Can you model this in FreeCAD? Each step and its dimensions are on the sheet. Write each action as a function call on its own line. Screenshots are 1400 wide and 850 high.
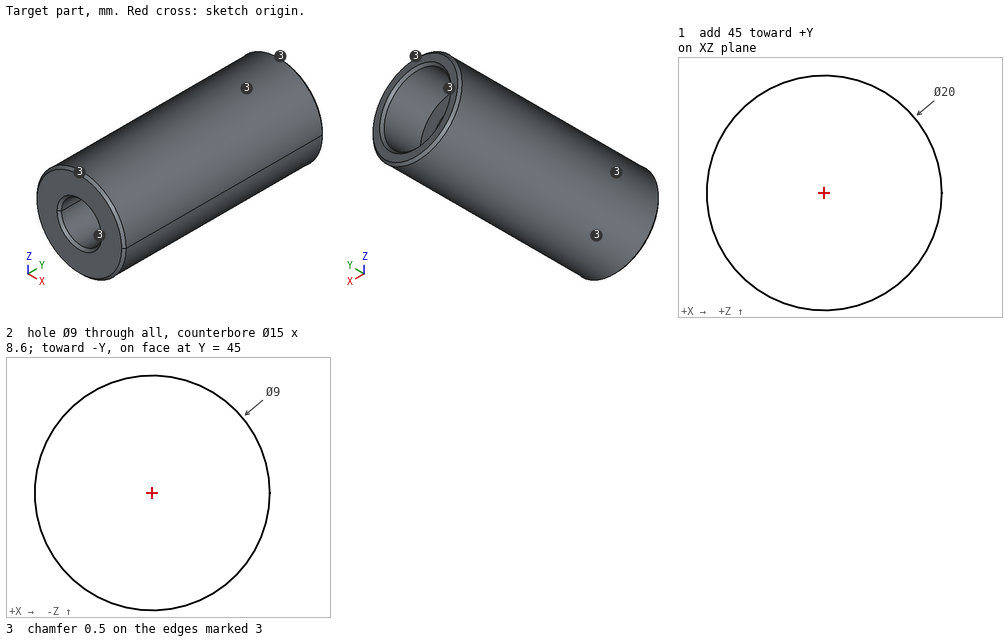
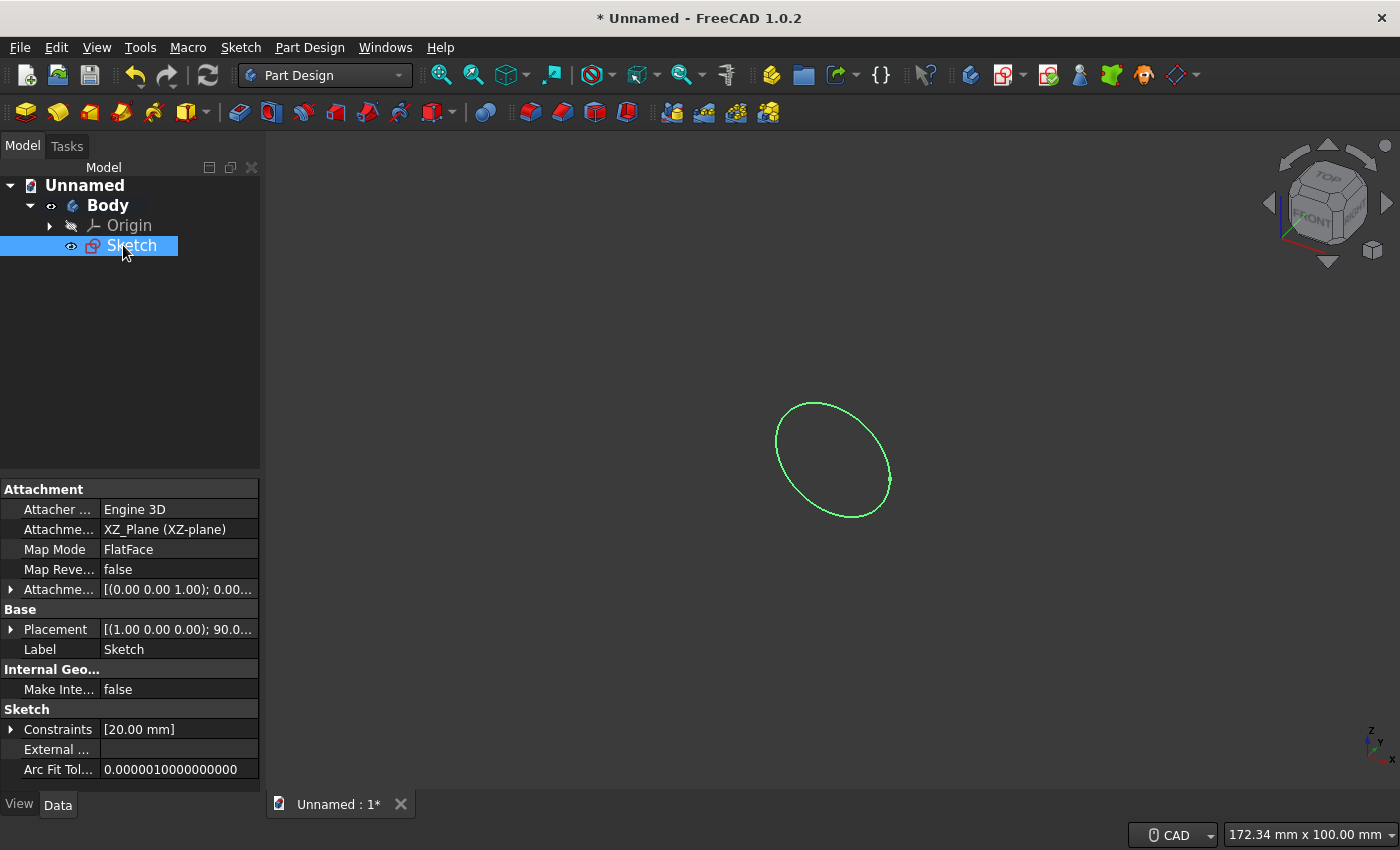
click(26, 112)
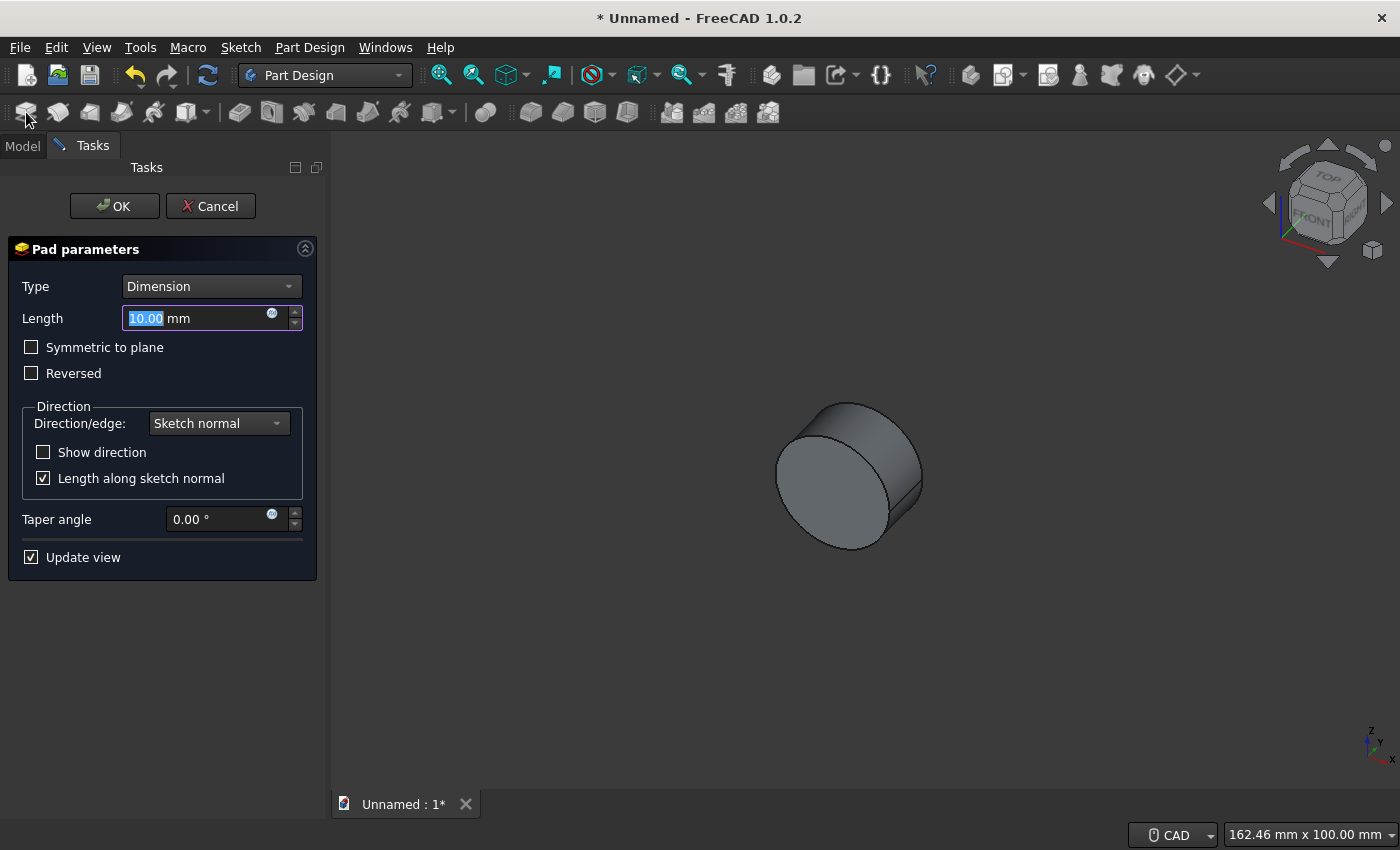
text(45)
key(Tab)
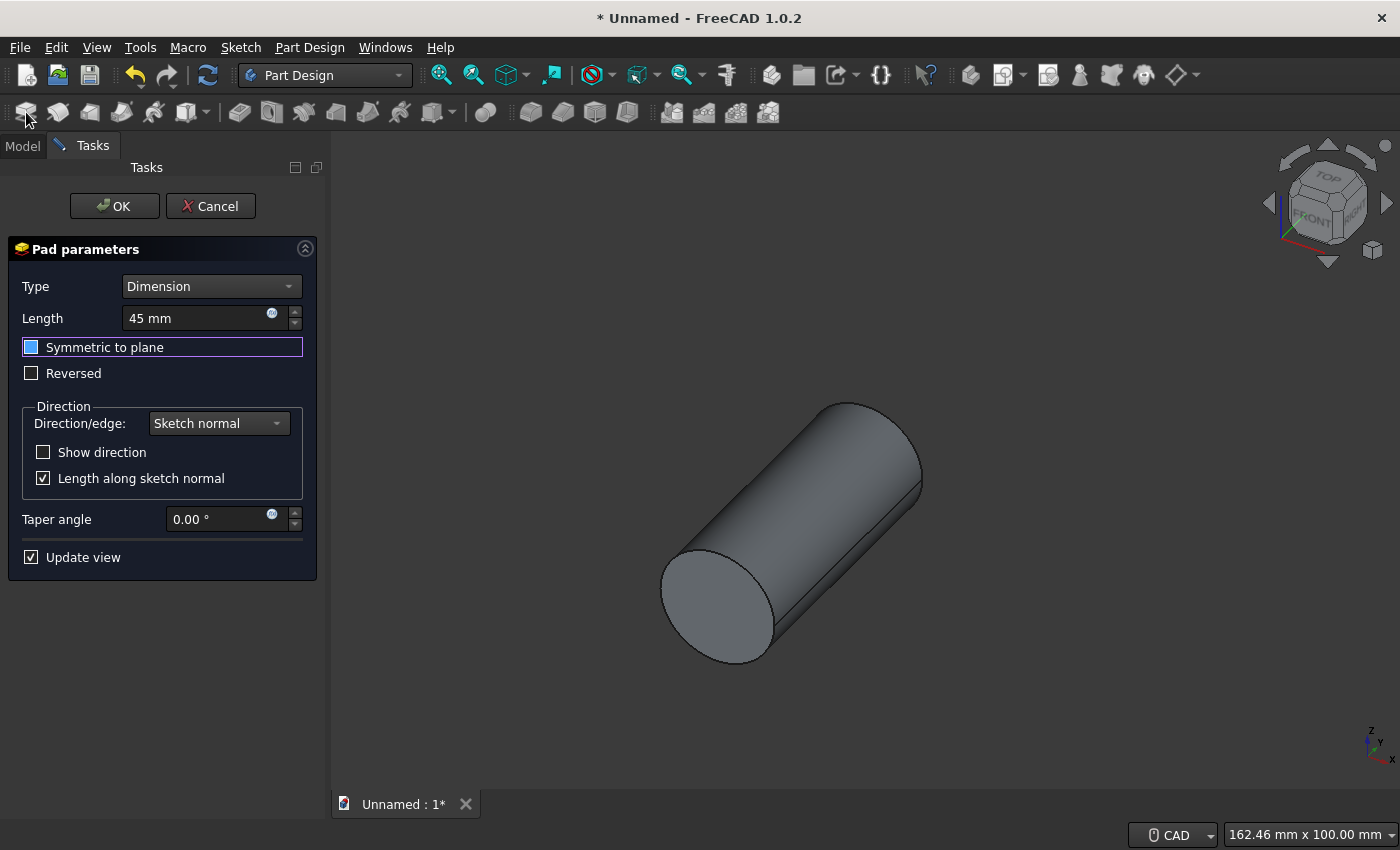
click(30, 373)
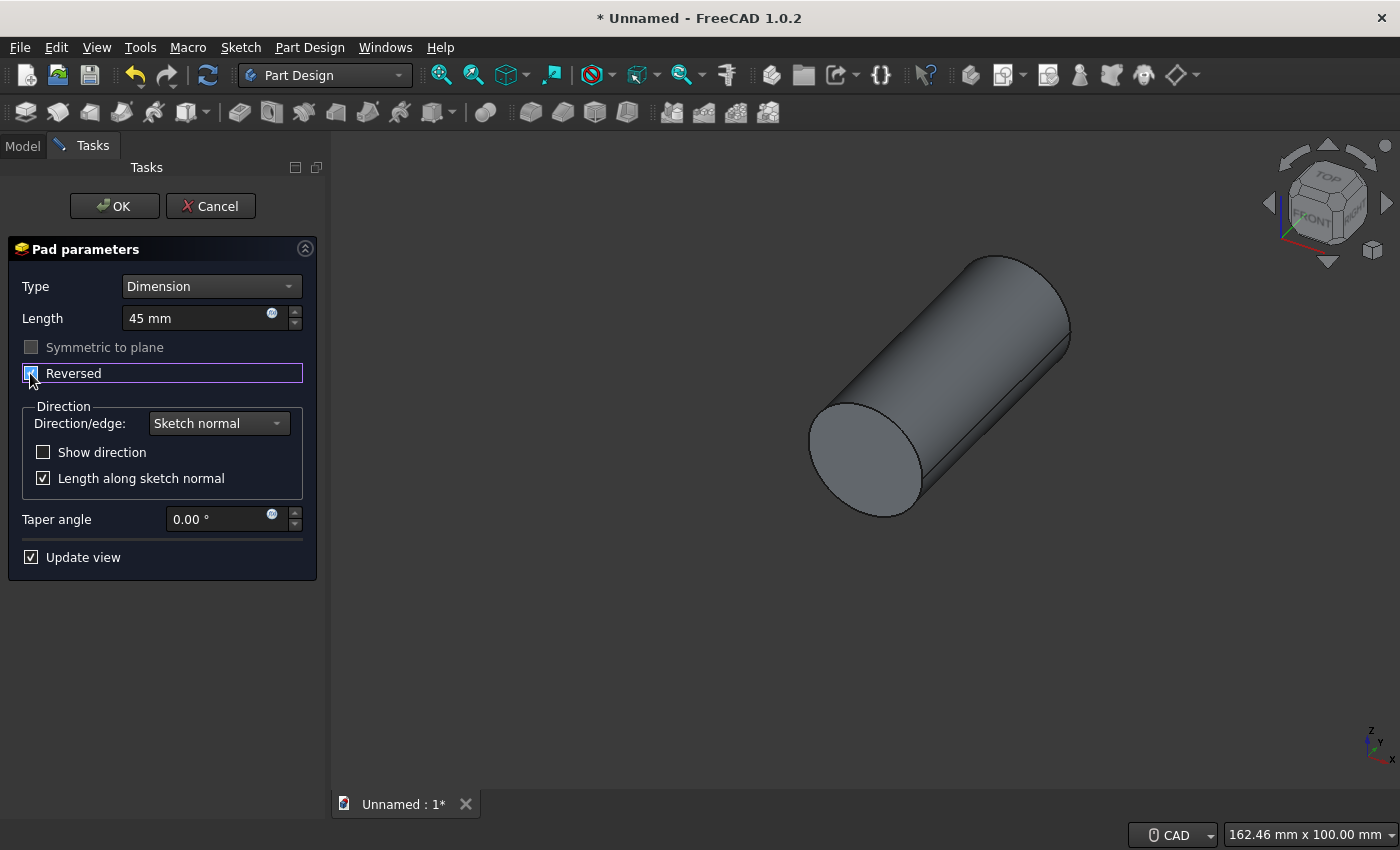
click(115, 206)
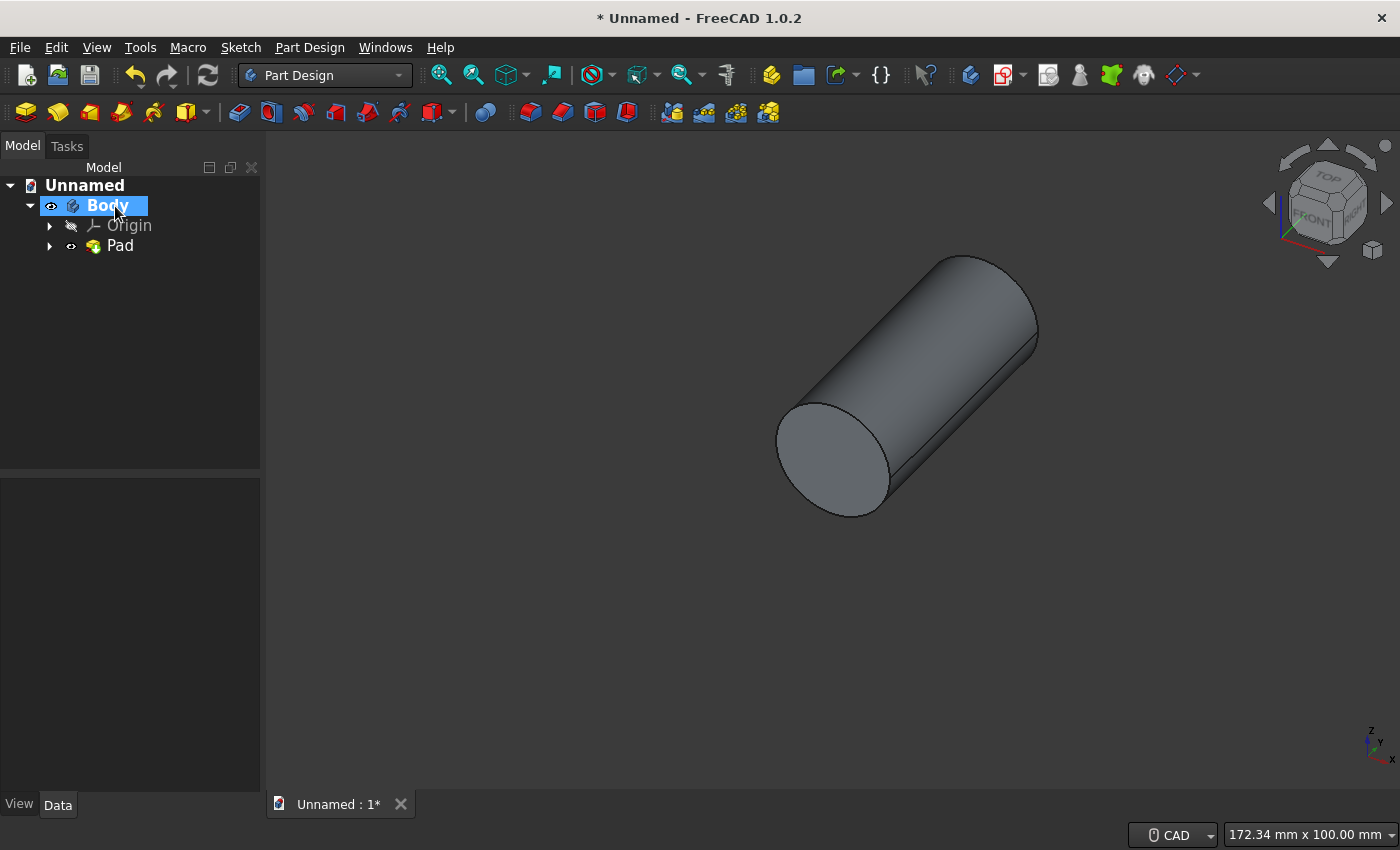
key(v)
key(f)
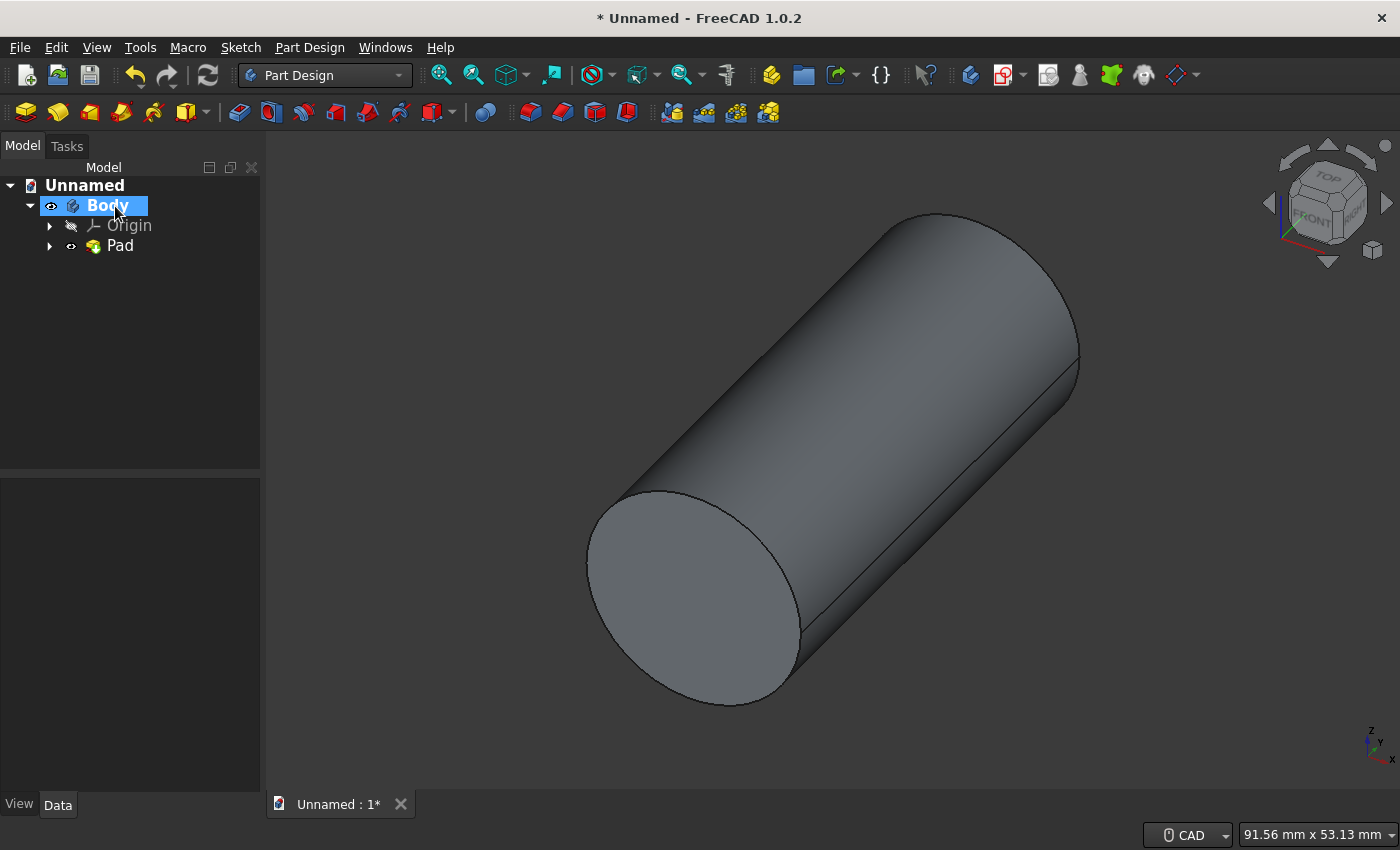
key(4)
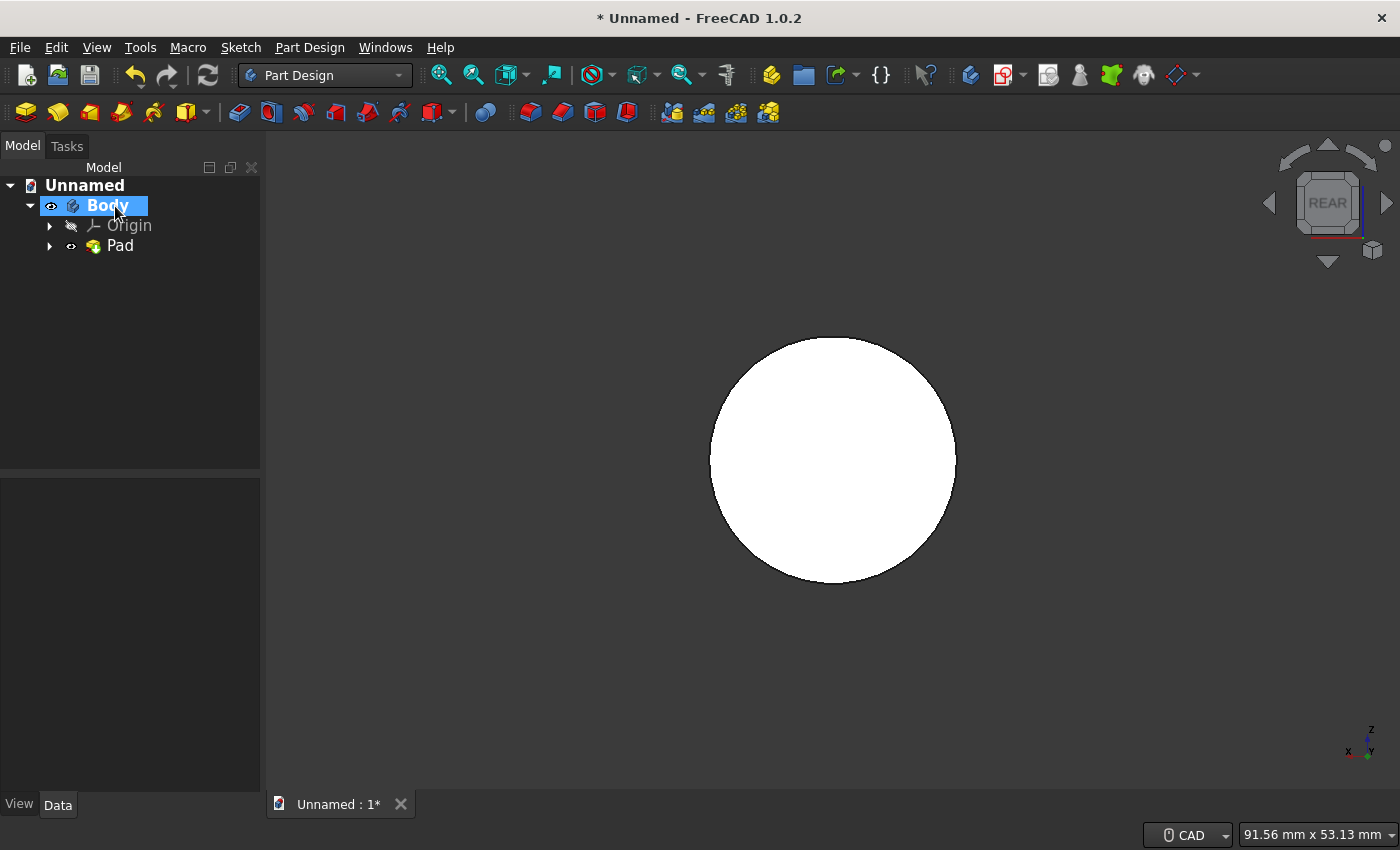
click(442, 76)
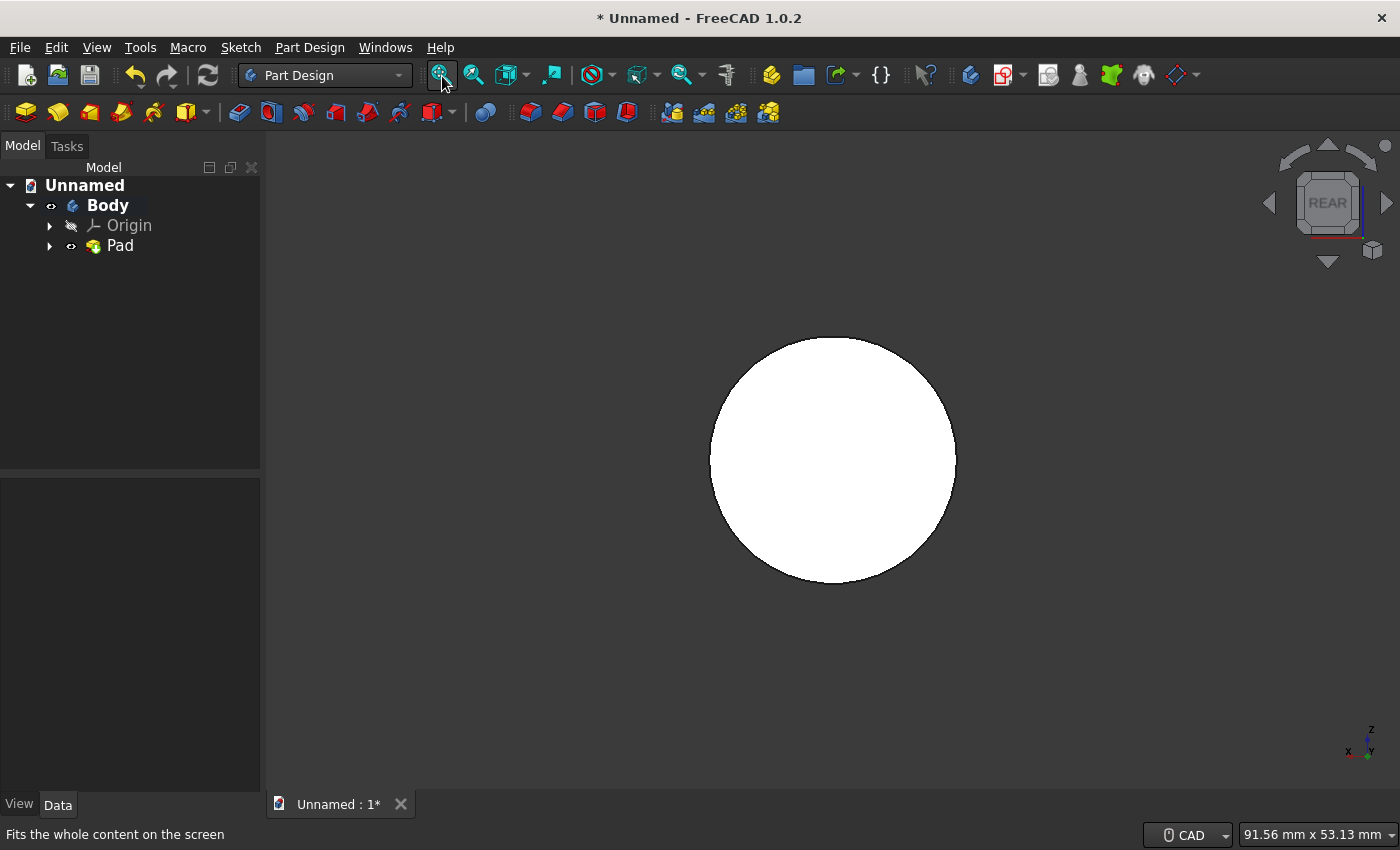
click(833, 459)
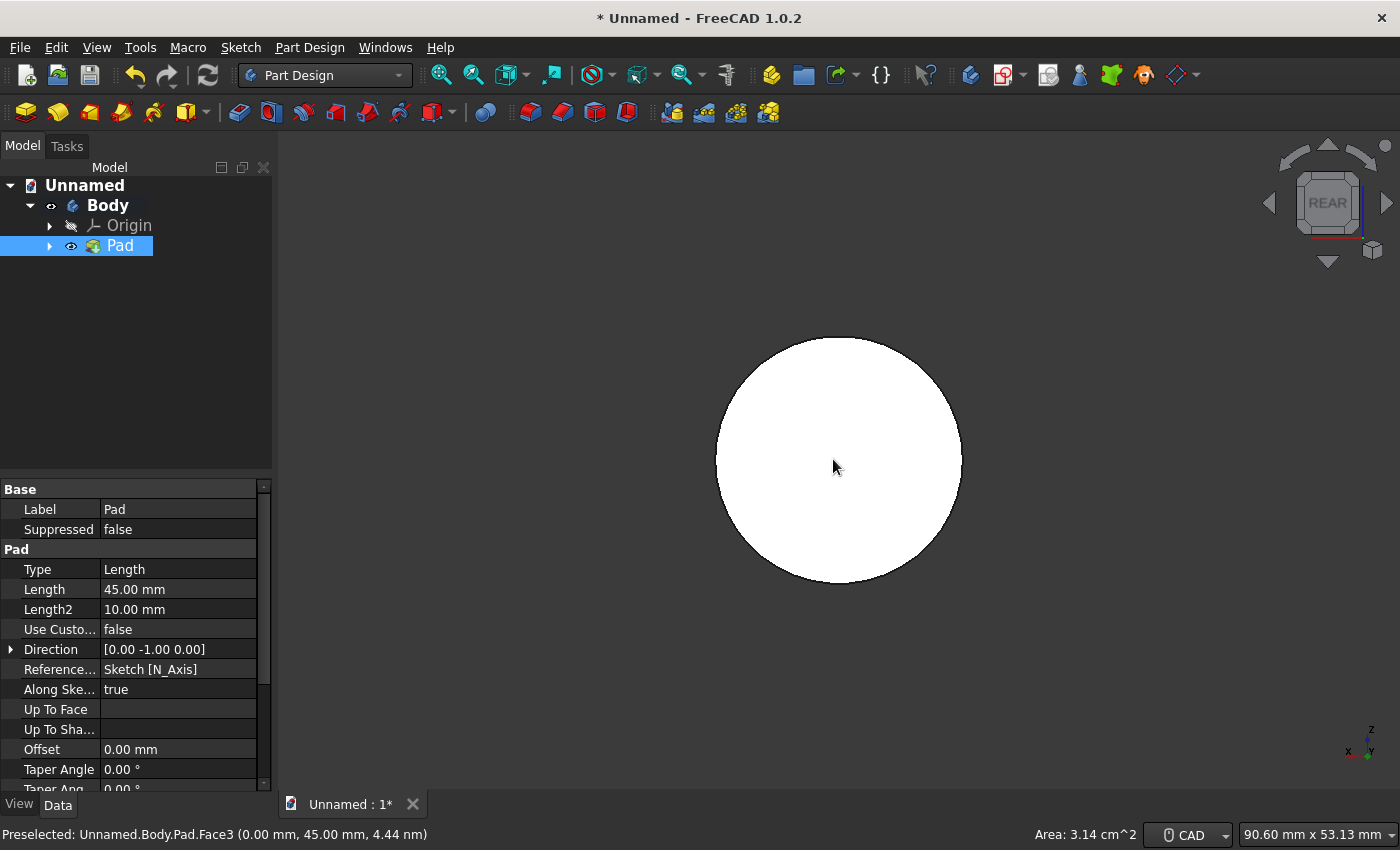
click(1004, 76)